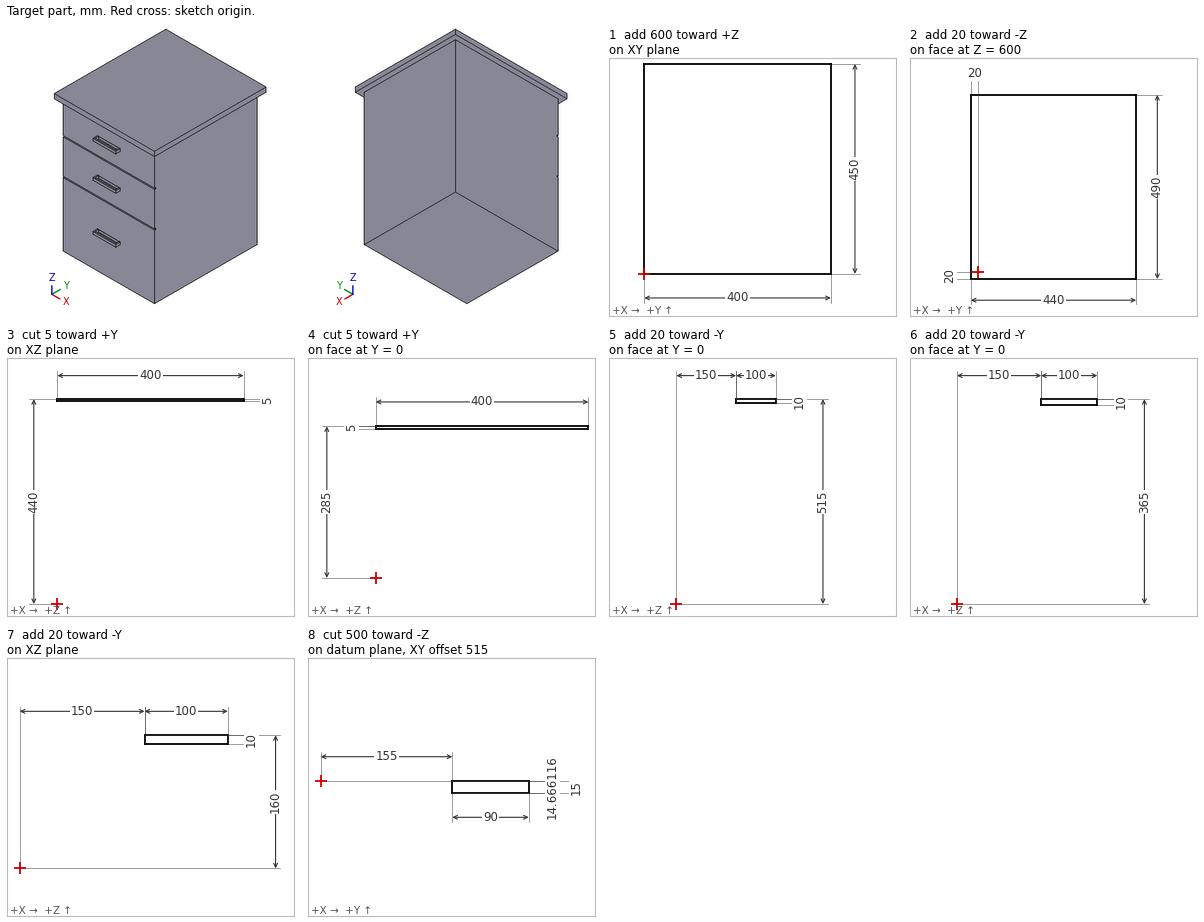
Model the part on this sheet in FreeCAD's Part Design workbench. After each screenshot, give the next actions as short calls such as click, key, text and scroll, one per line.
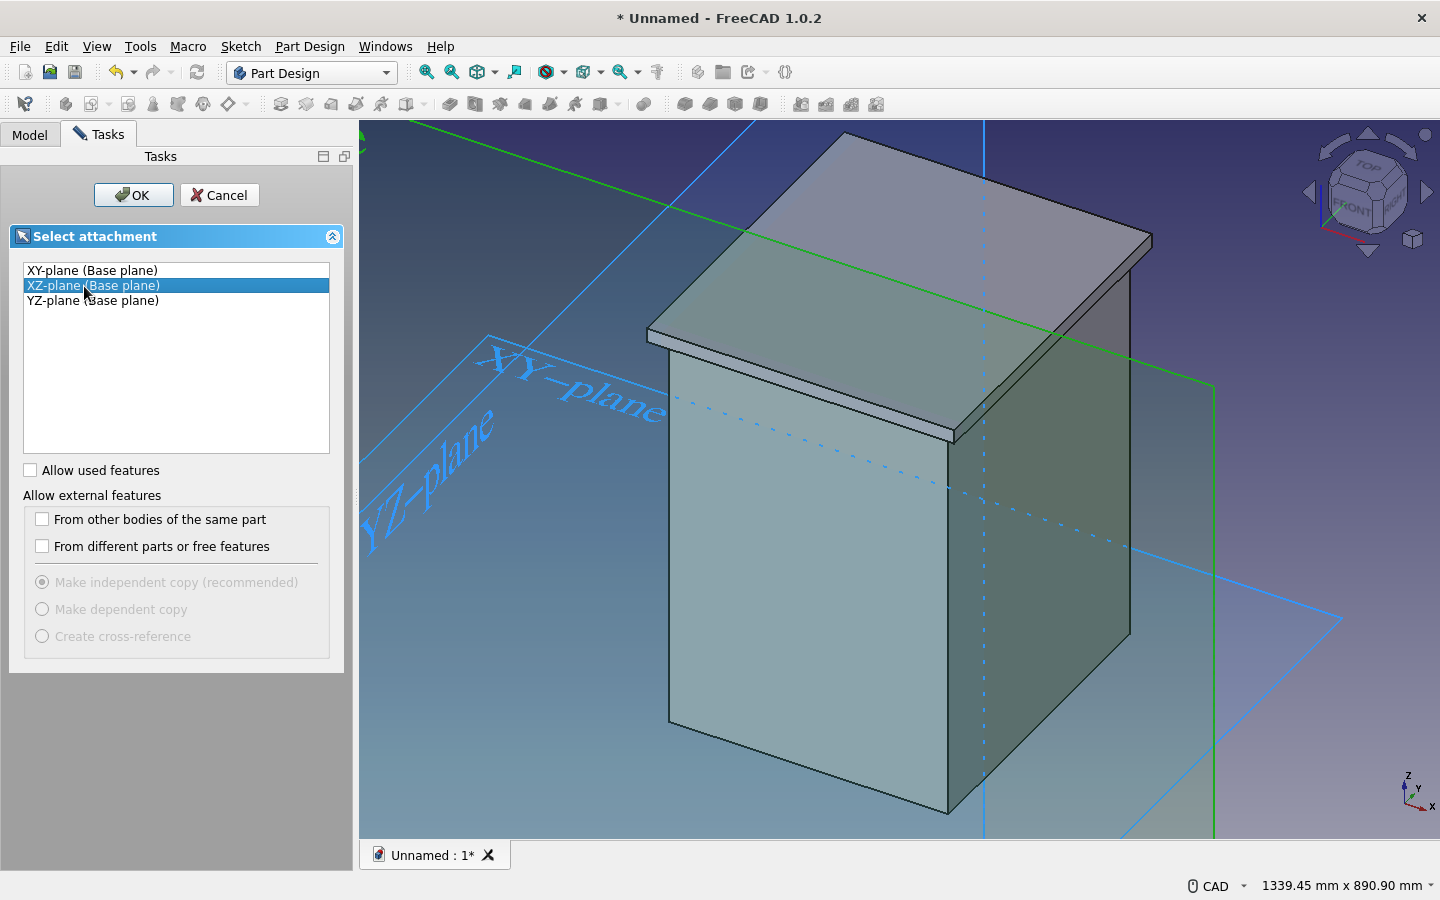
click(134, 195)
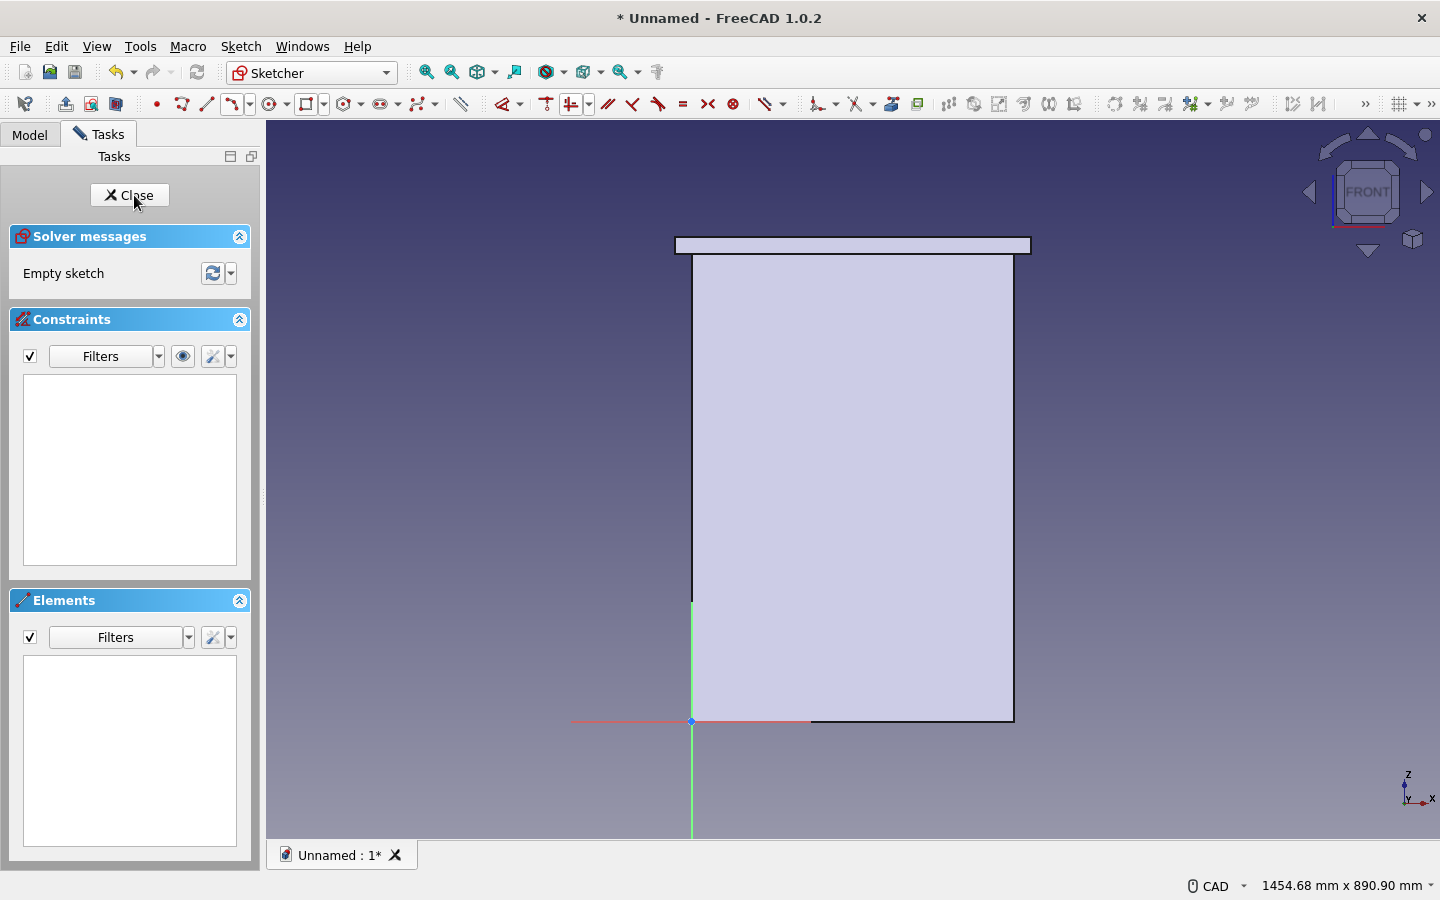
click(116, 104)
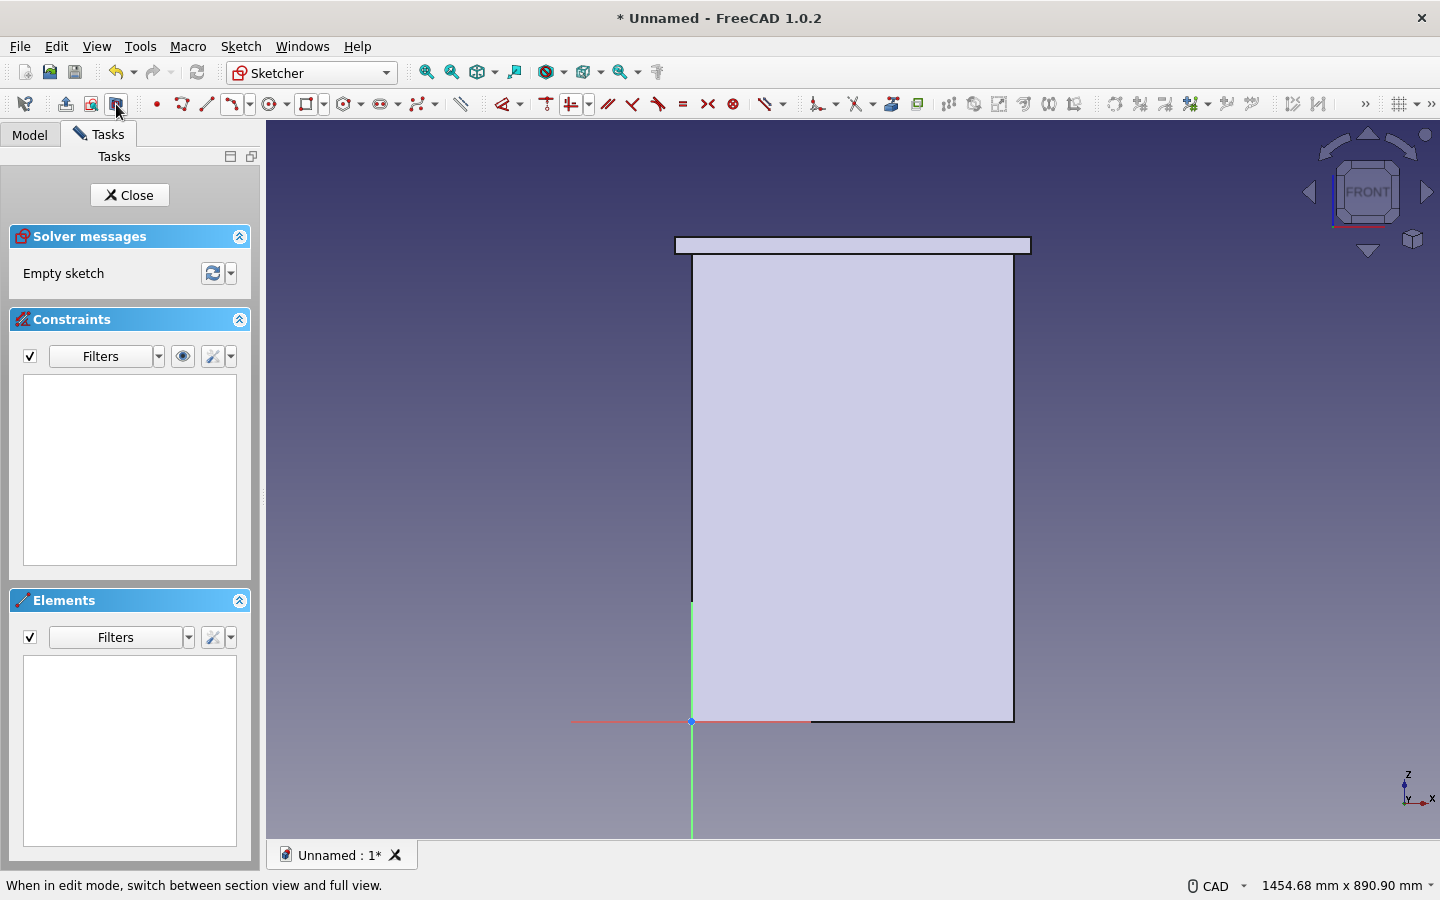
click(306, 104)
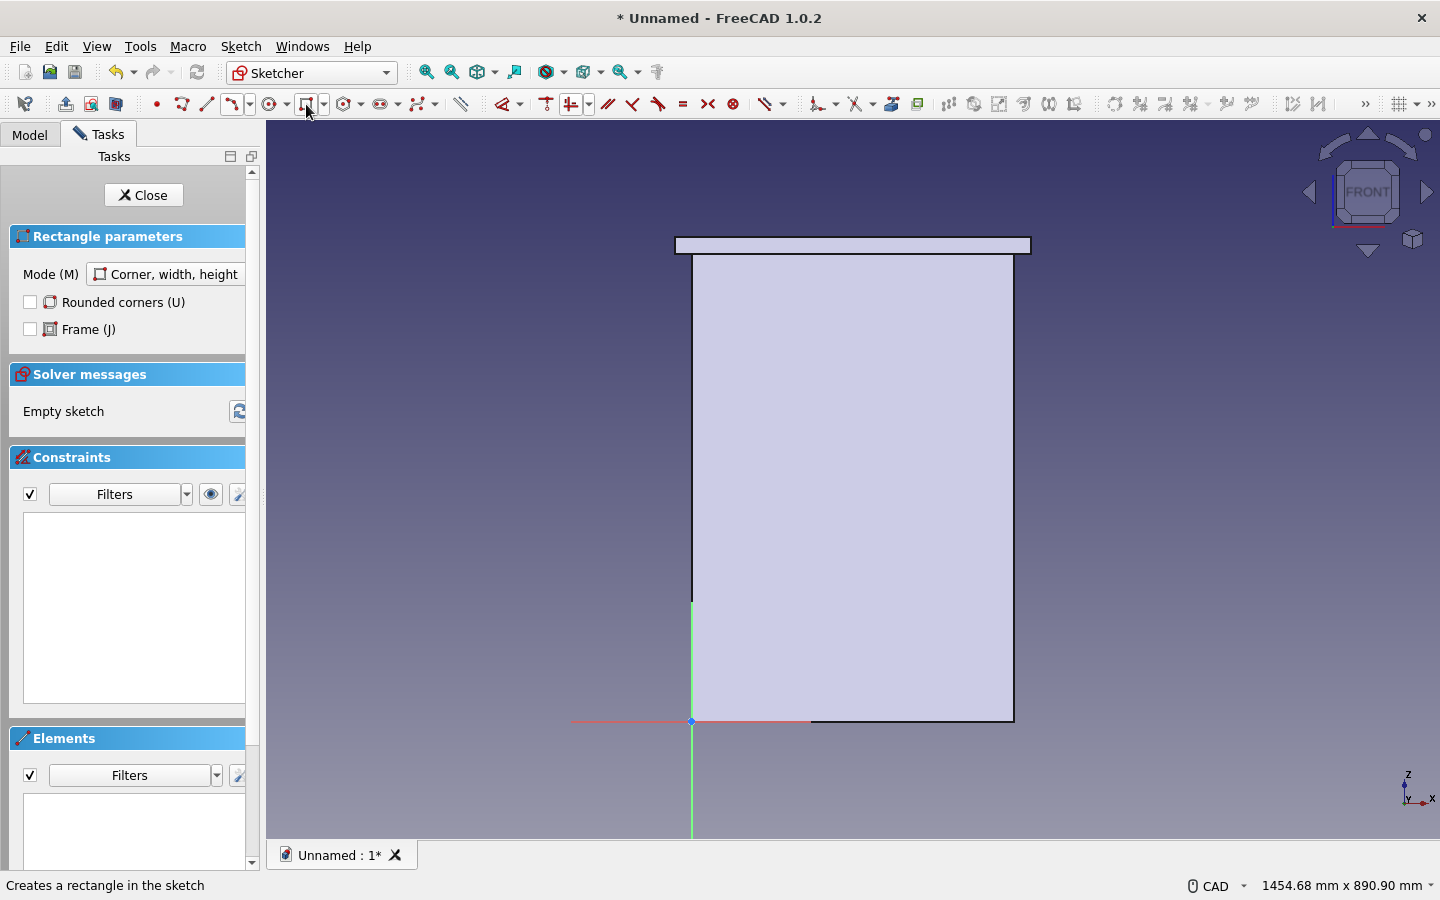
scroll(692, 367, up, 7)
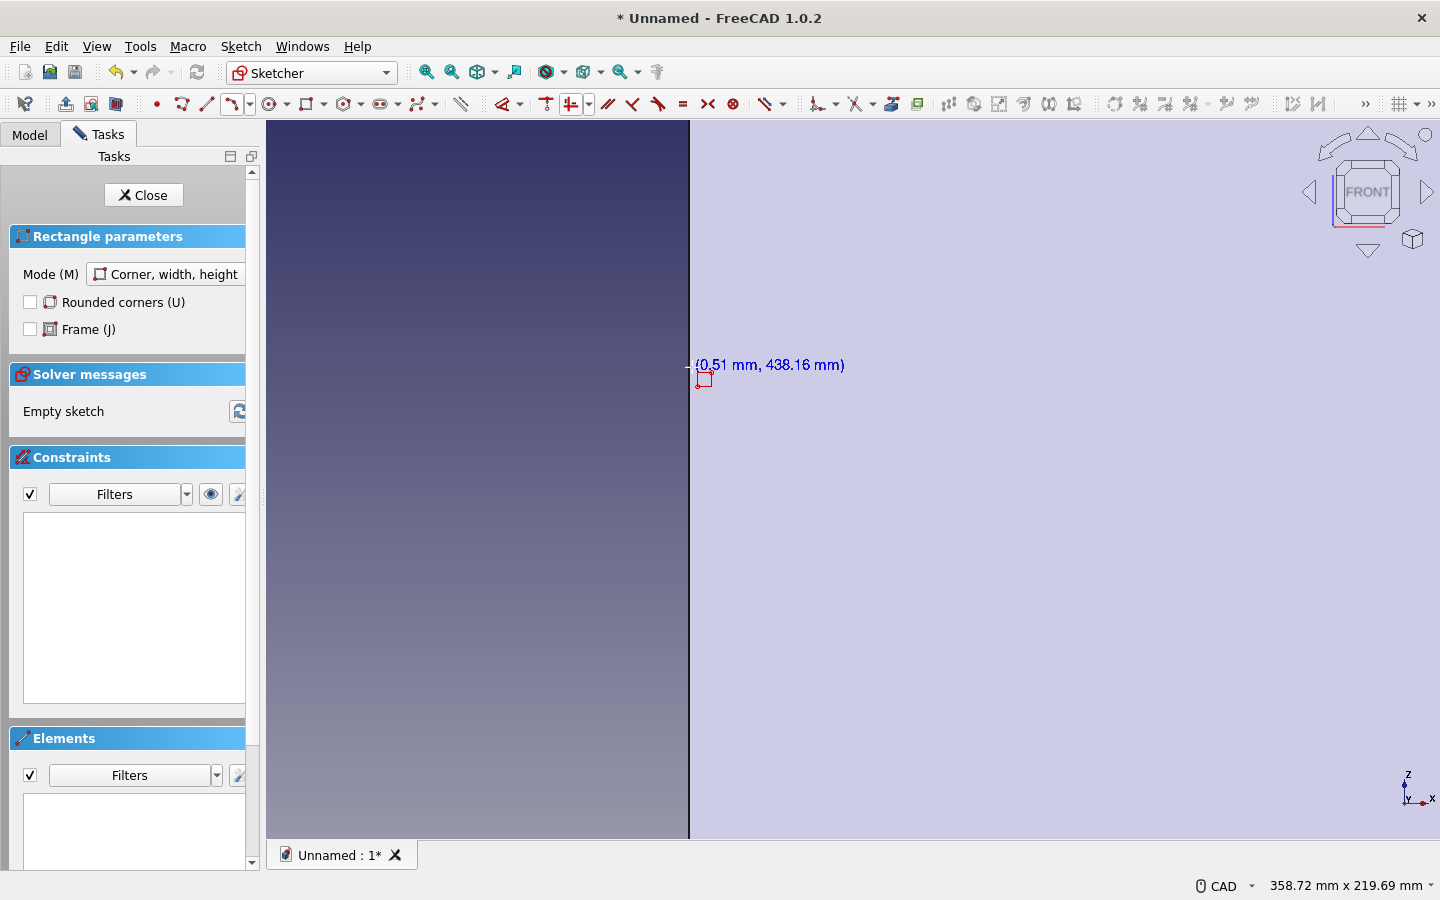
scroll(543, 219, down, 6)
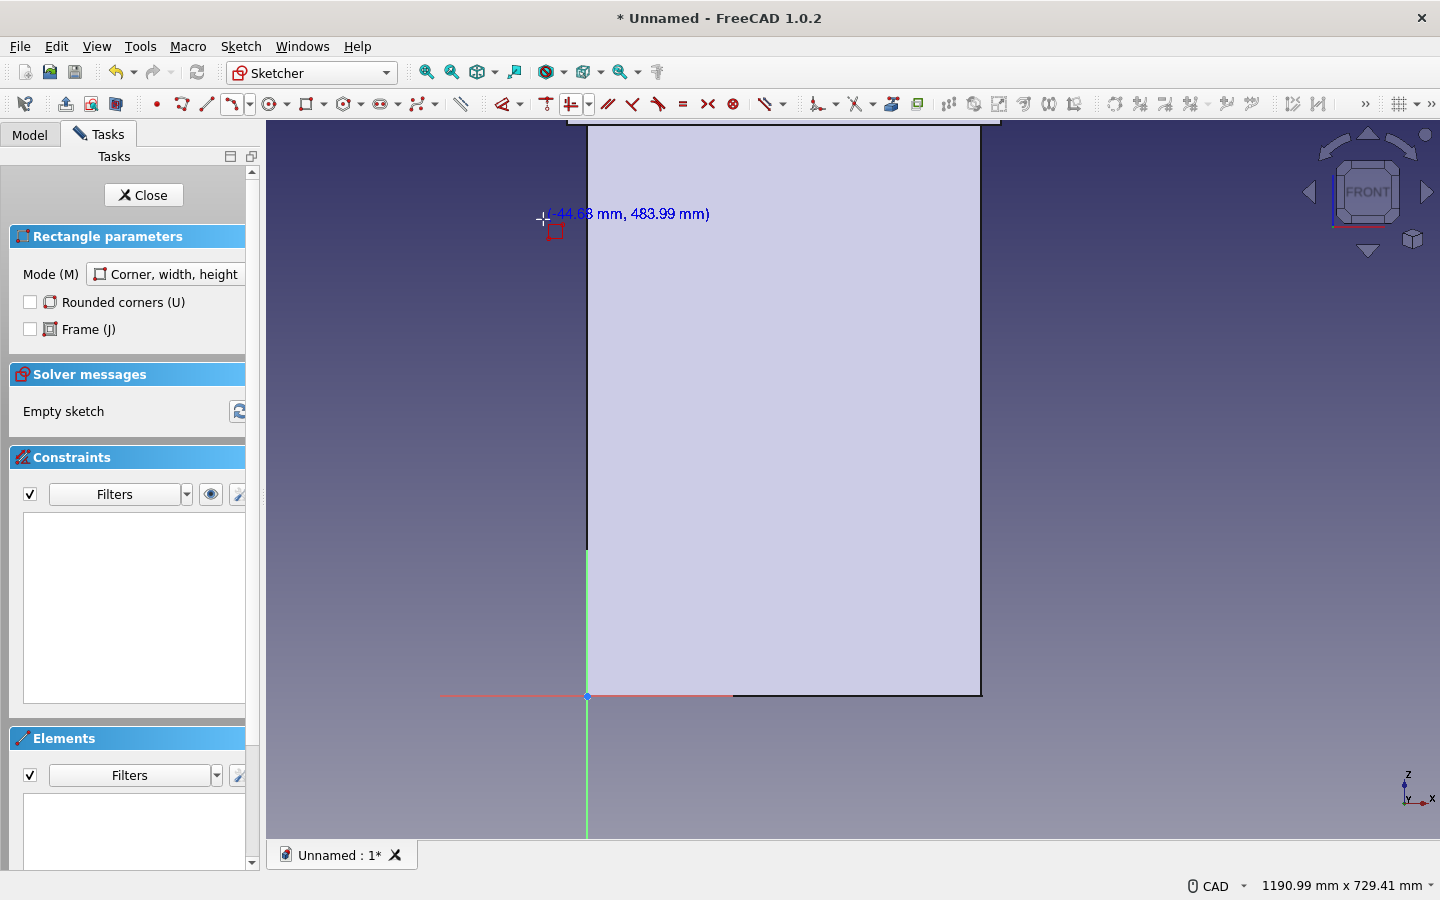
click(587, 263)
move(982, 268)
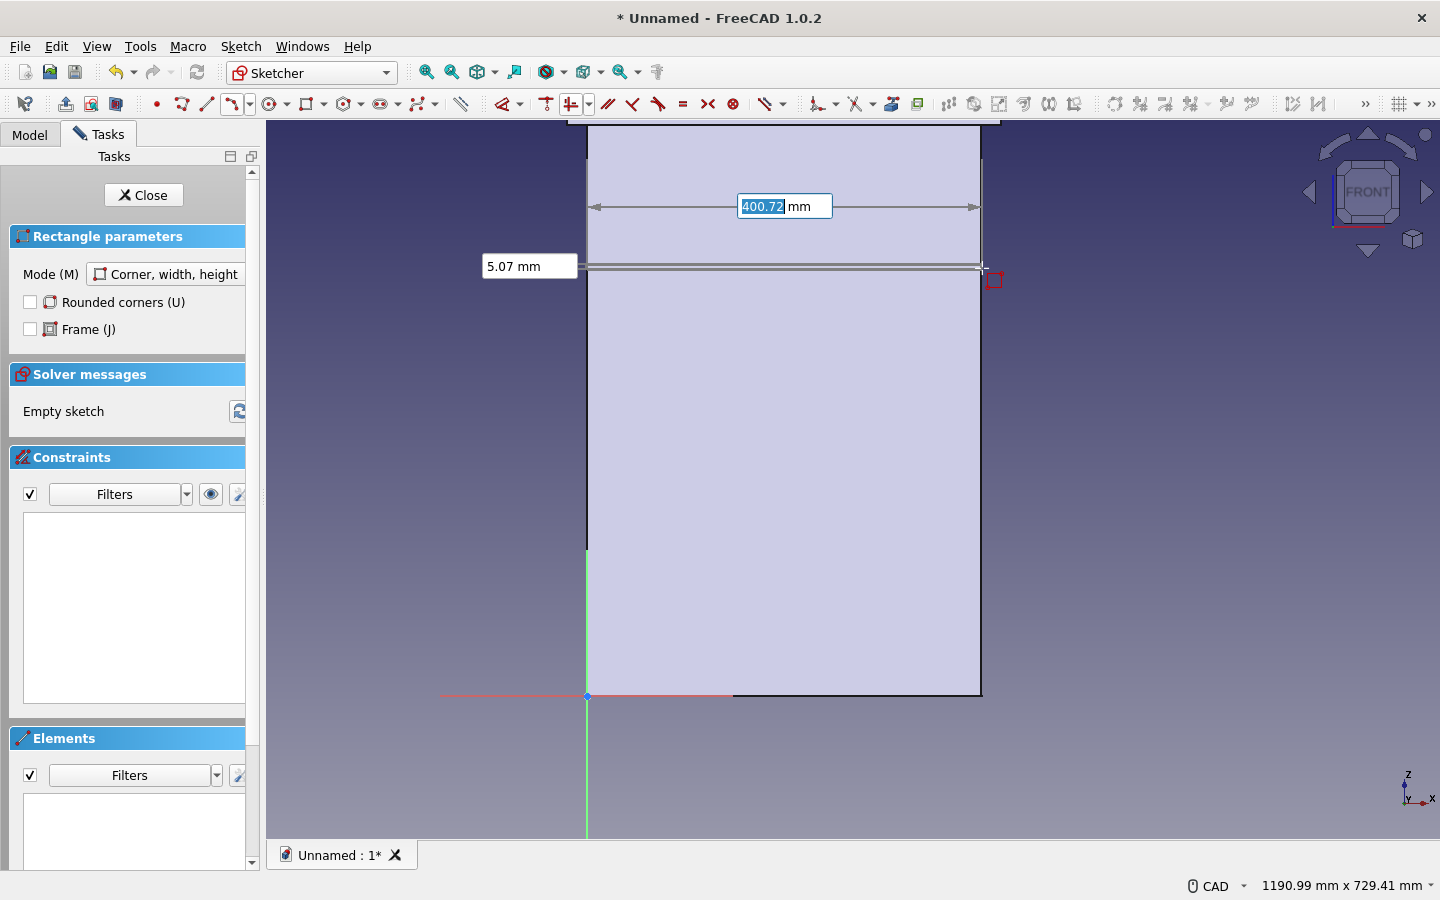
text(400)
key(Tab)
text(5)
key(Return)
key(Escape)